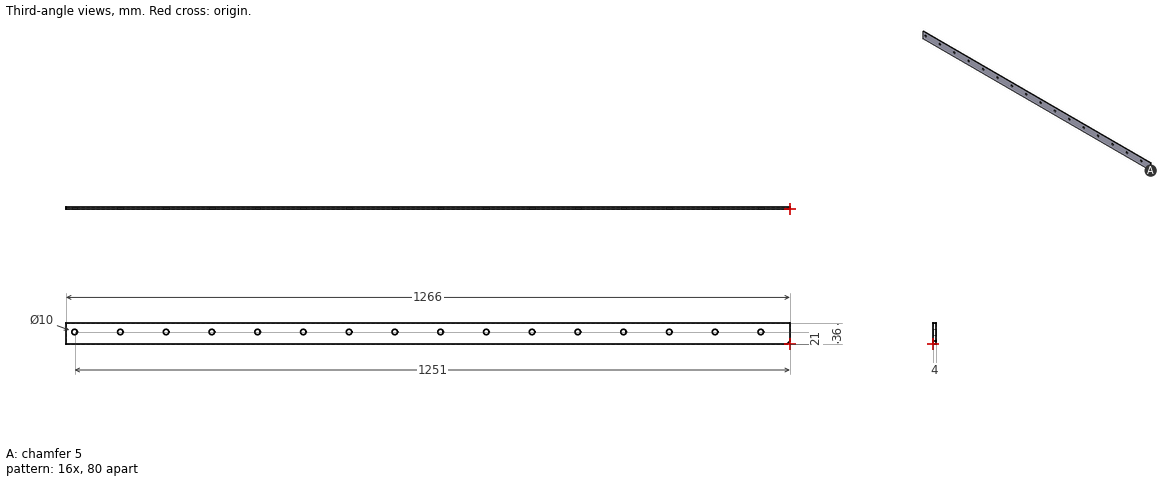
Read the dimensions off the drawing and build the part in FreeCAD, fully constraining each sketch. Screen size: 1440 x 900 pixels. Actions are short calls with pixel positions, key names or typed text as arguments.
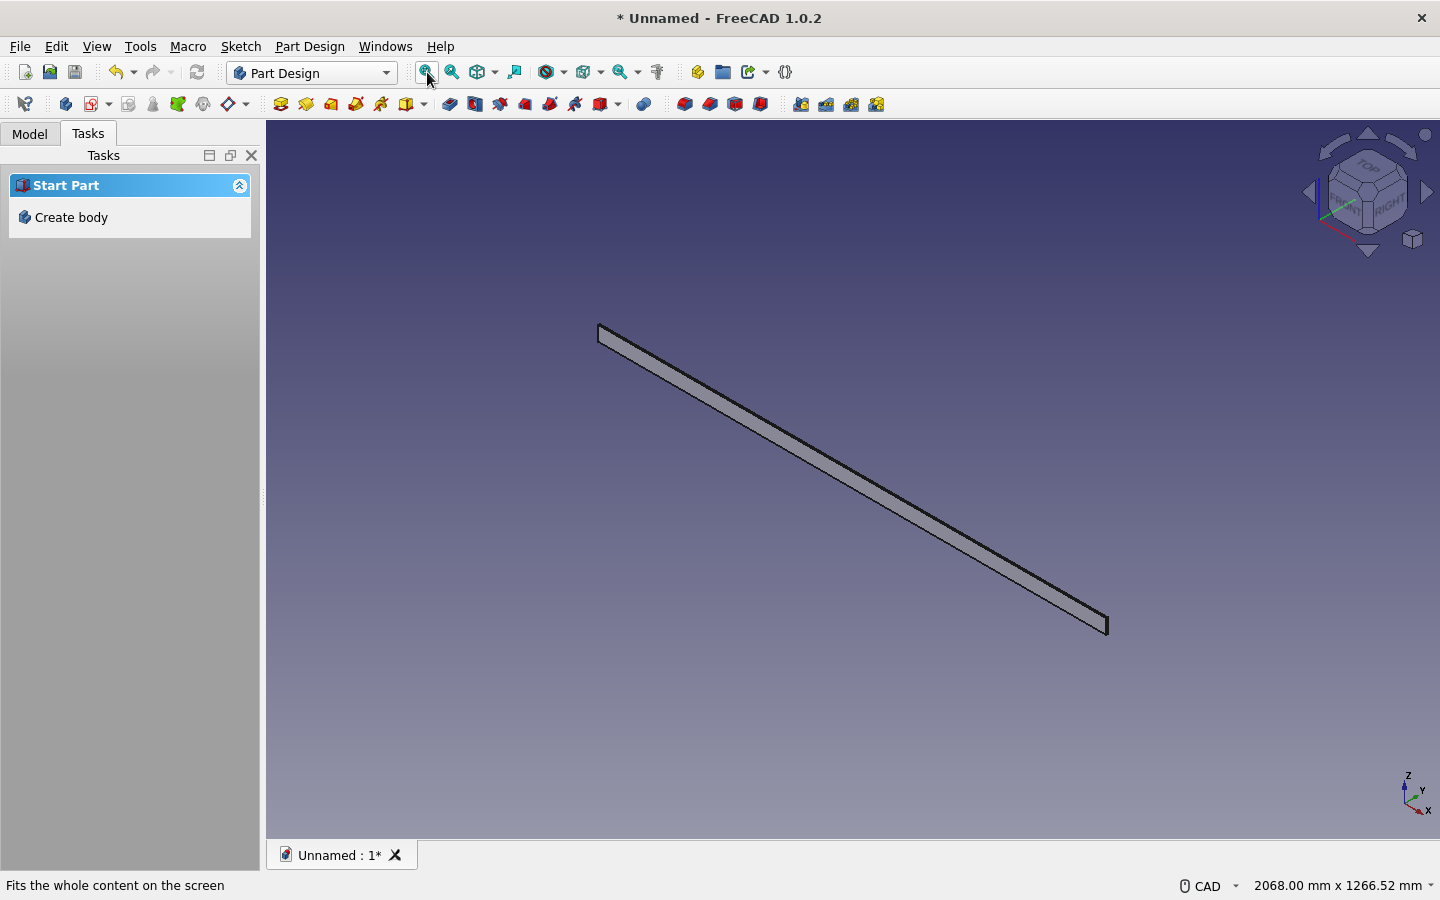
click(427, 72)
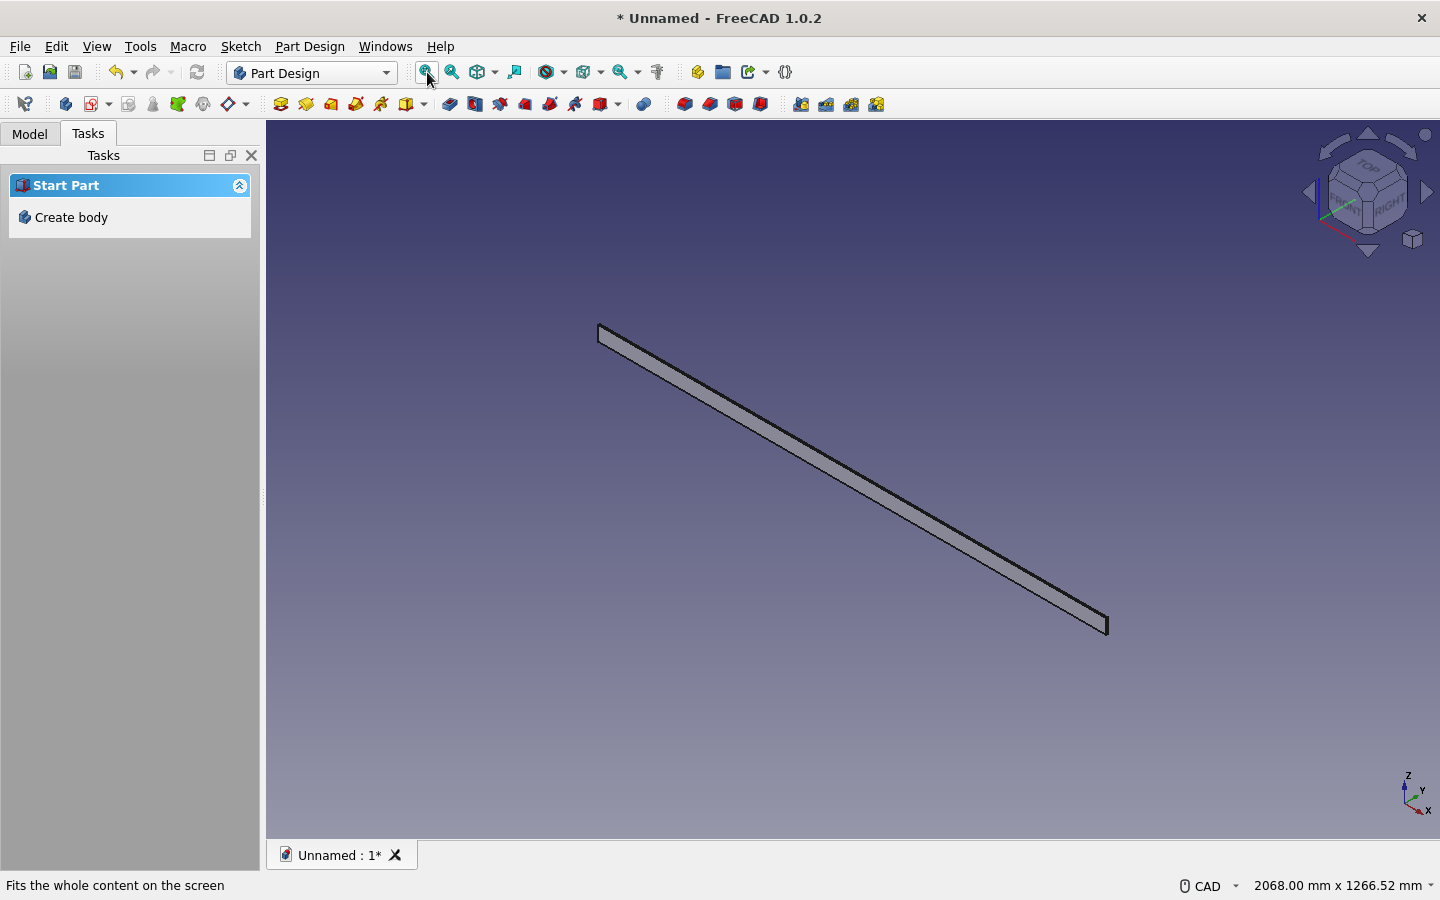
scroll(1107, 634, up, 15)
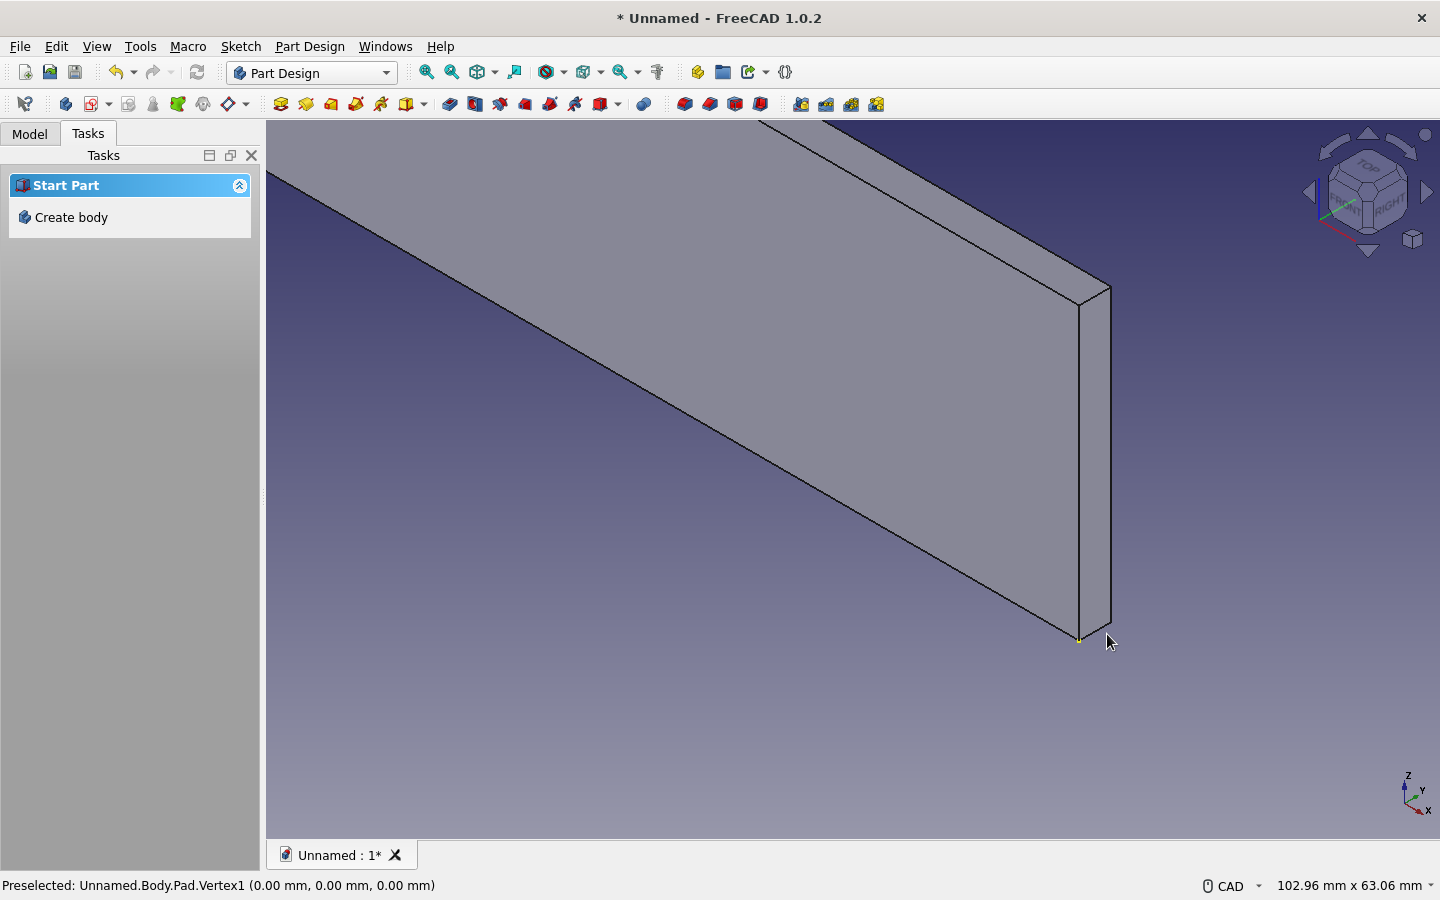
click(427, 72)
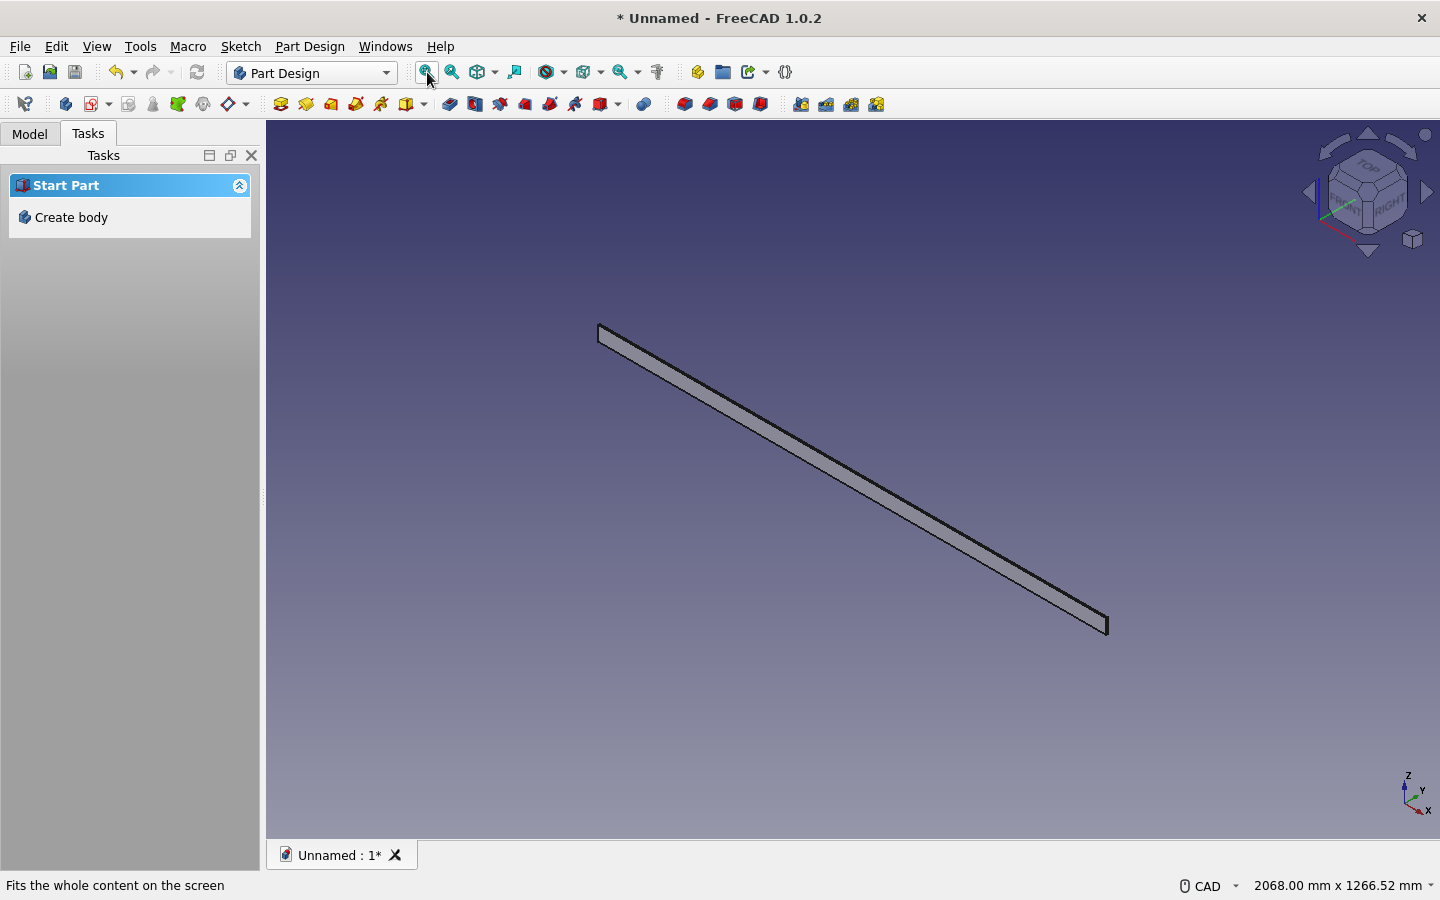
key(2)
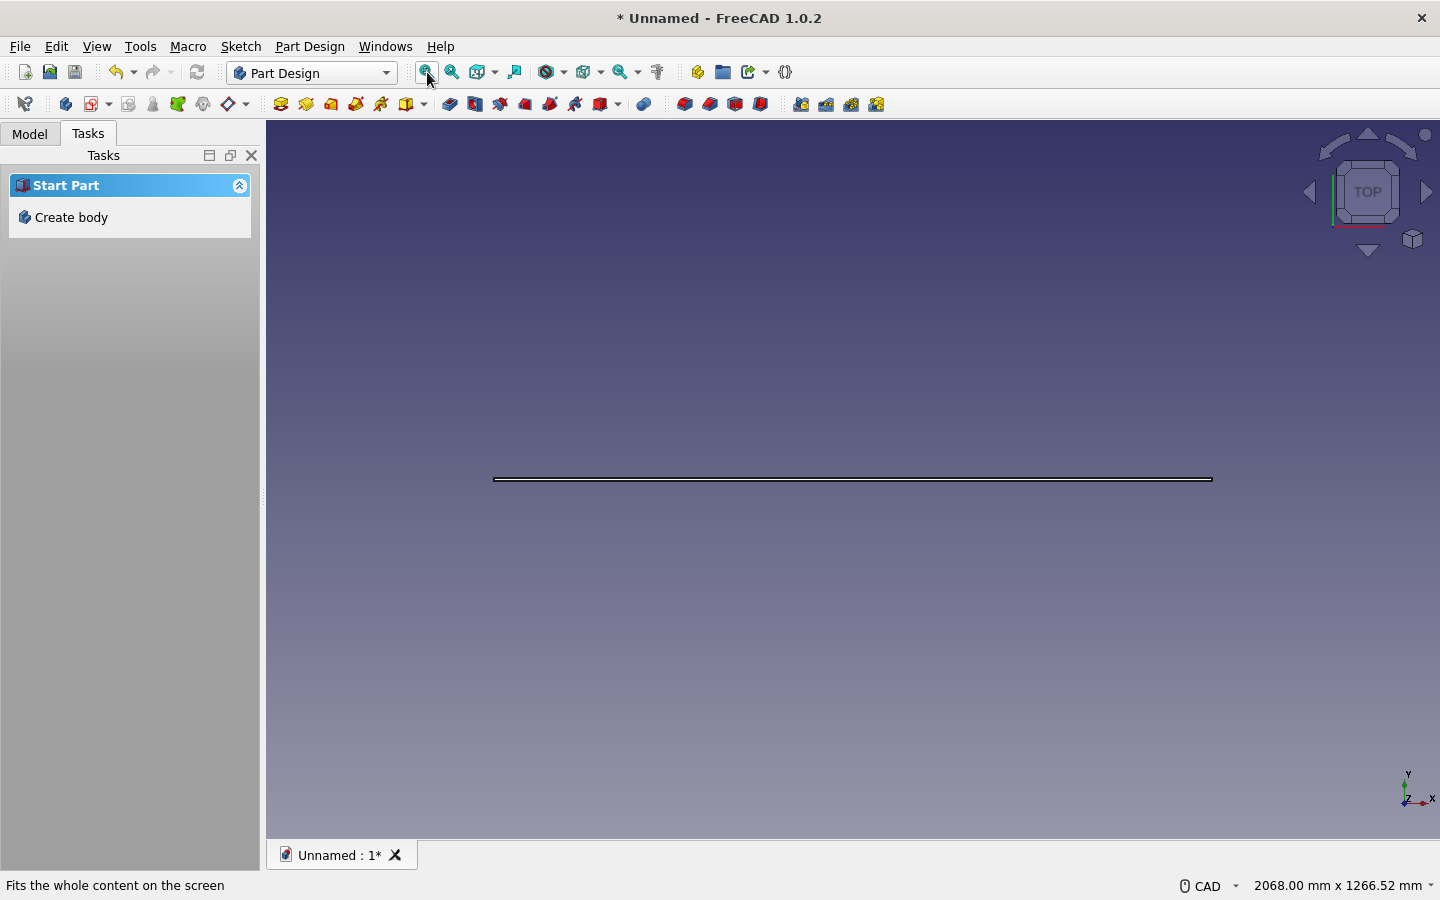
scroll(1212, 478, up, 15)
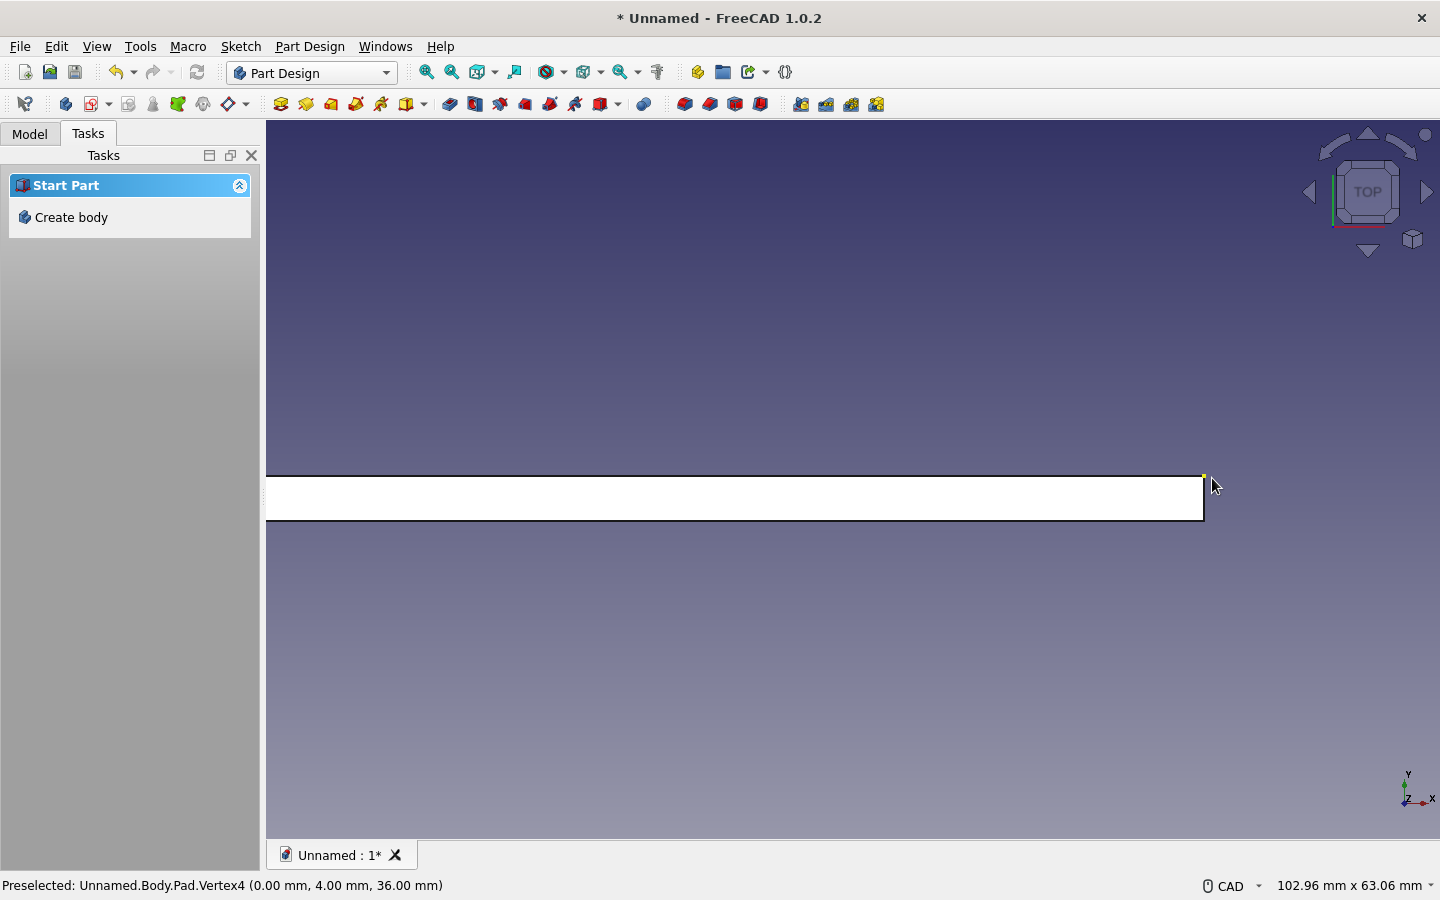
click(427, 72)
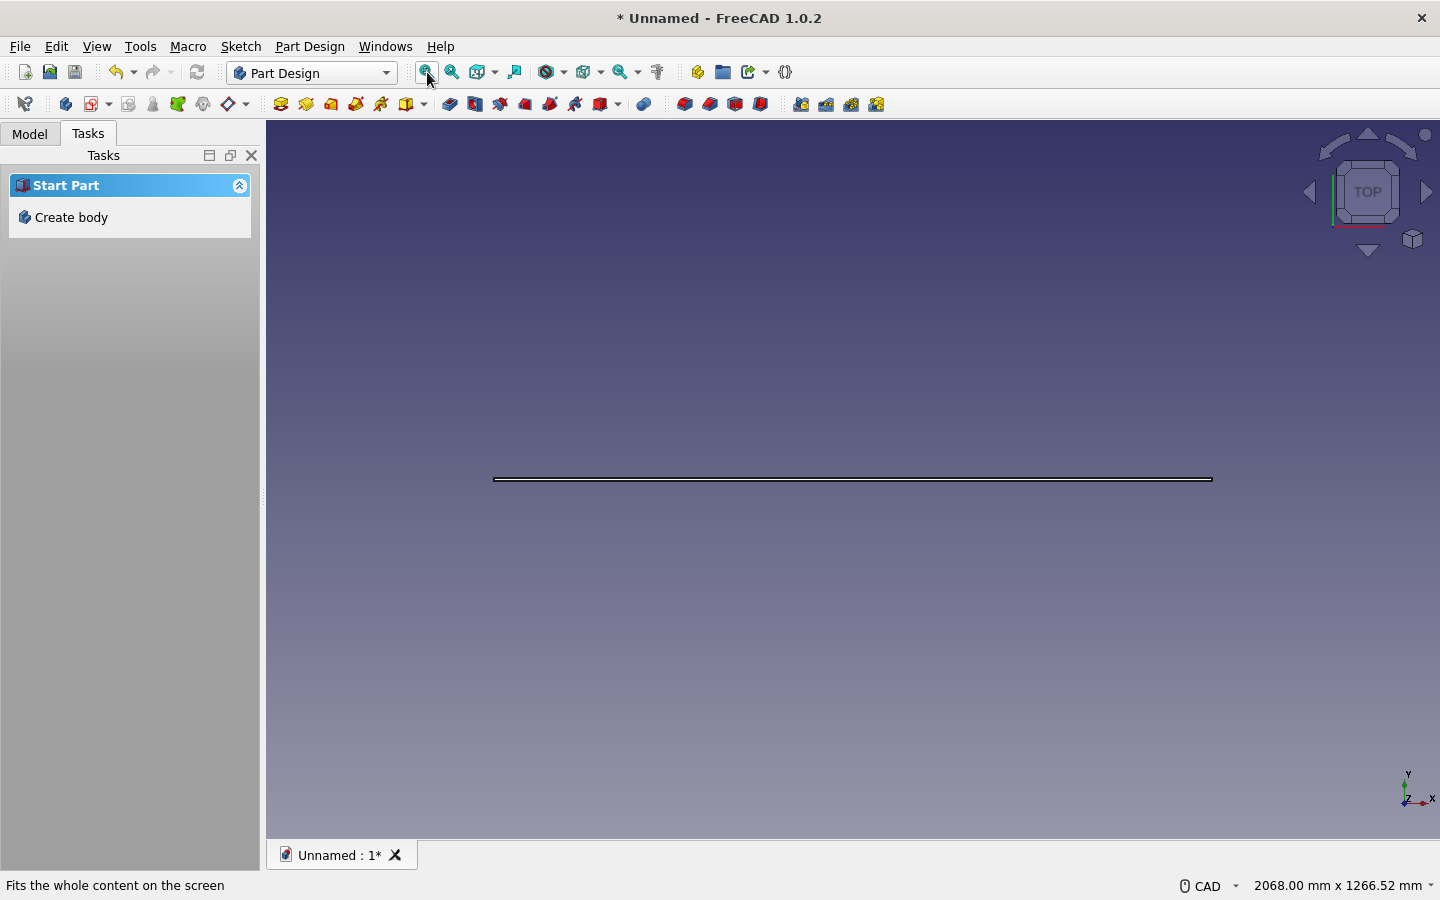
key(1)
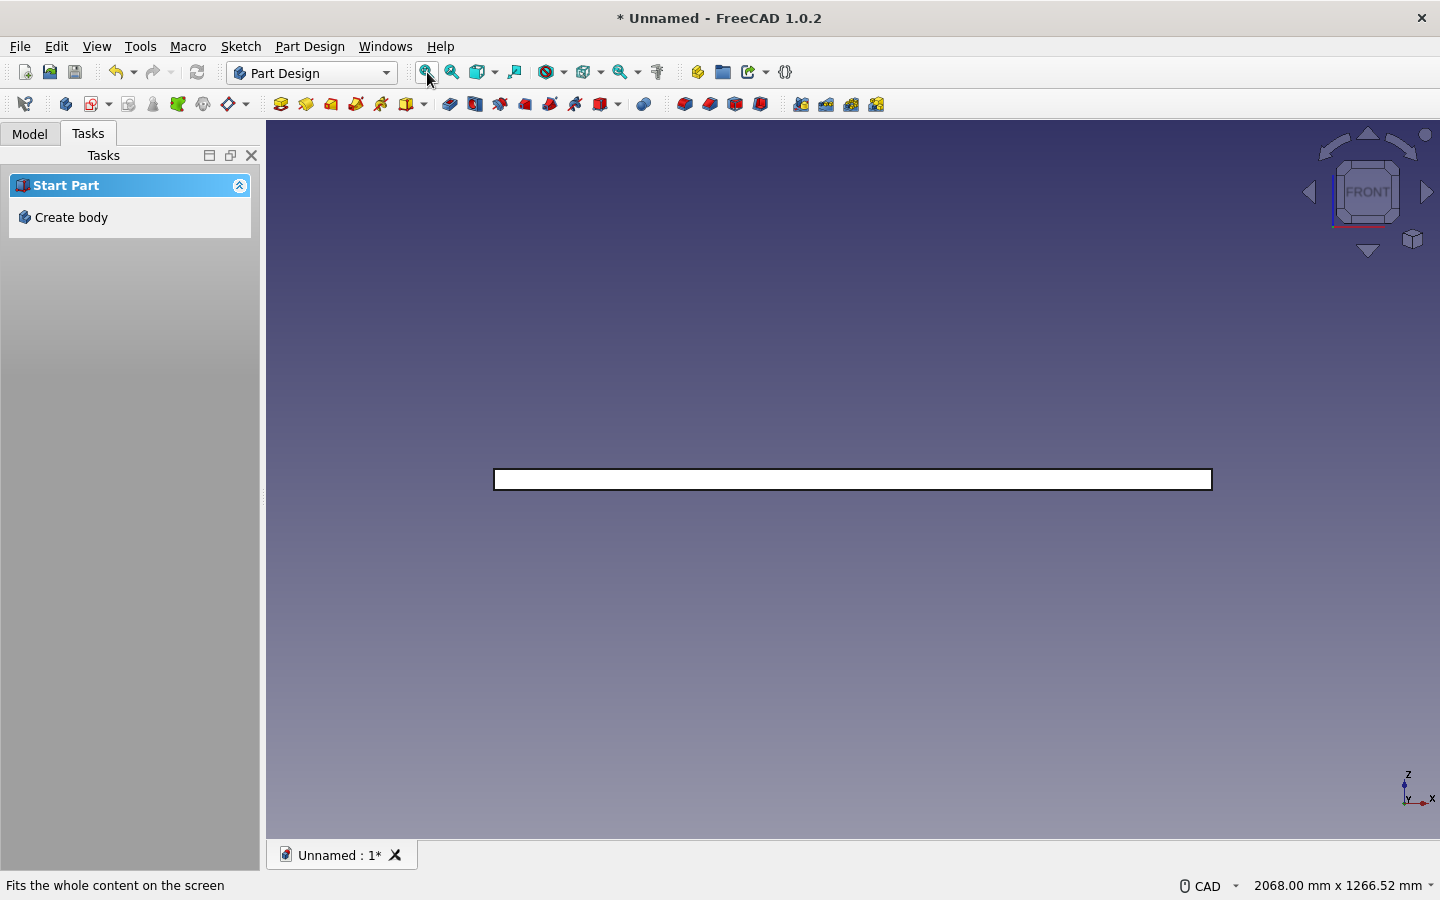
scroll(1212, 489, up, 15)